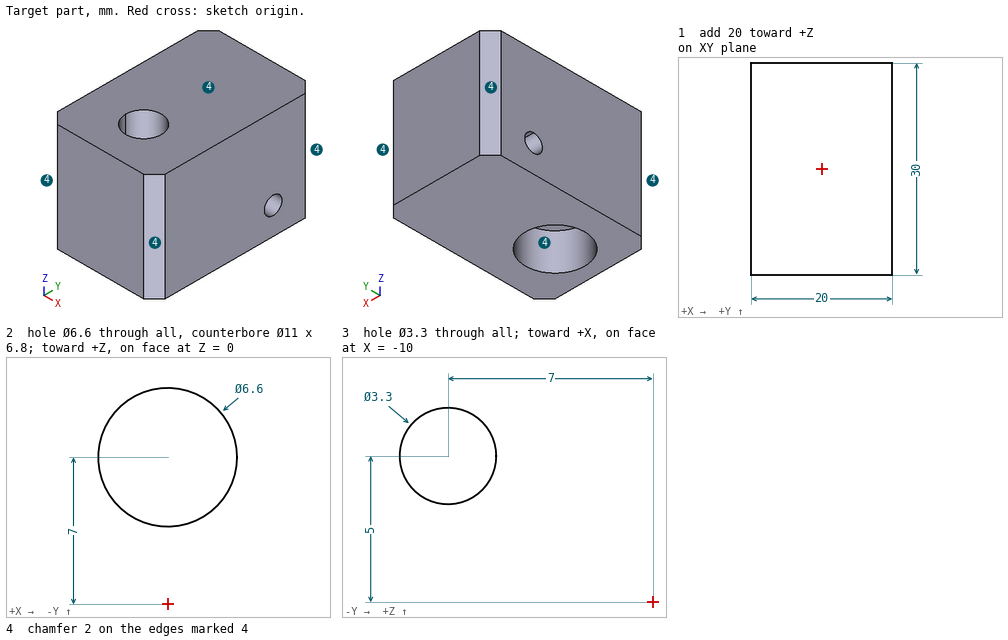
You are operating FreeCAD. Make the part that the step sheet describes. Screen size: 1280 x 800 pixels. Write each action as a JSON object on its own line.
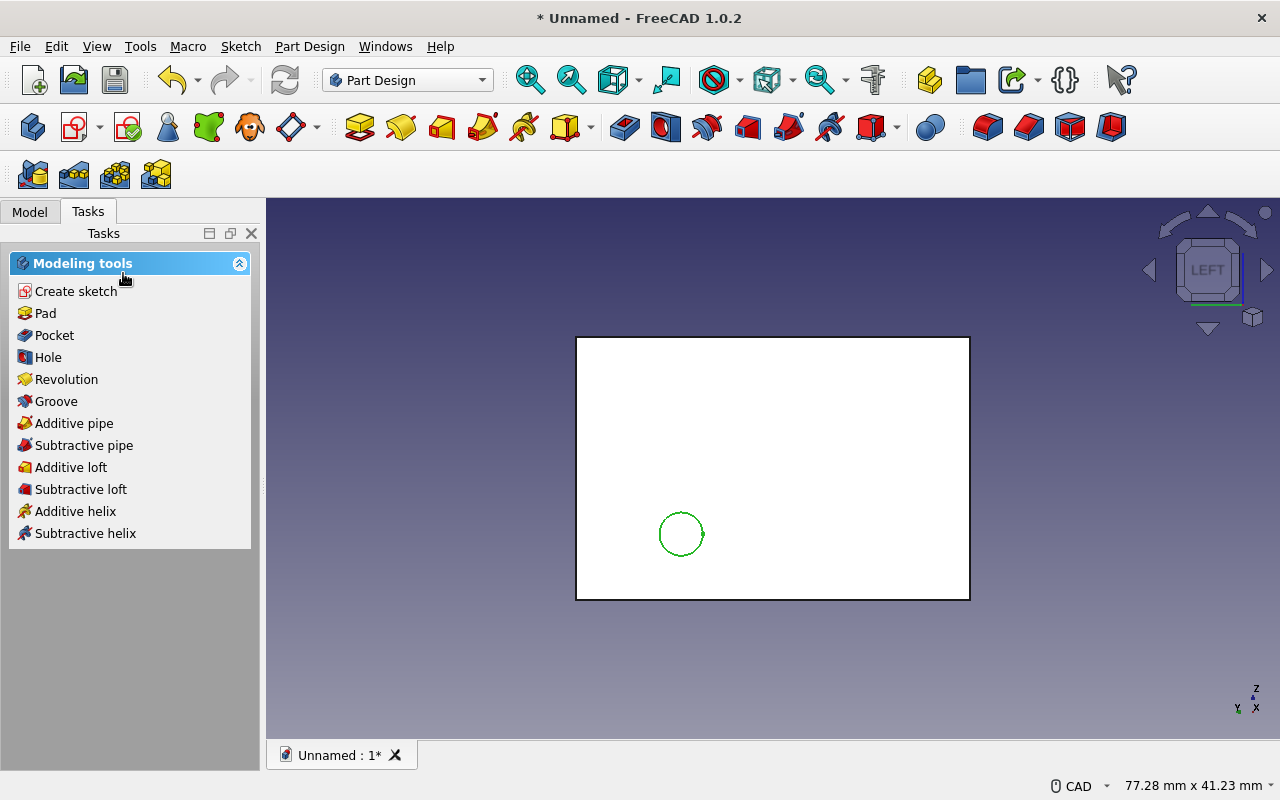
{"action": "left_click", "coordinate": [666, 128]}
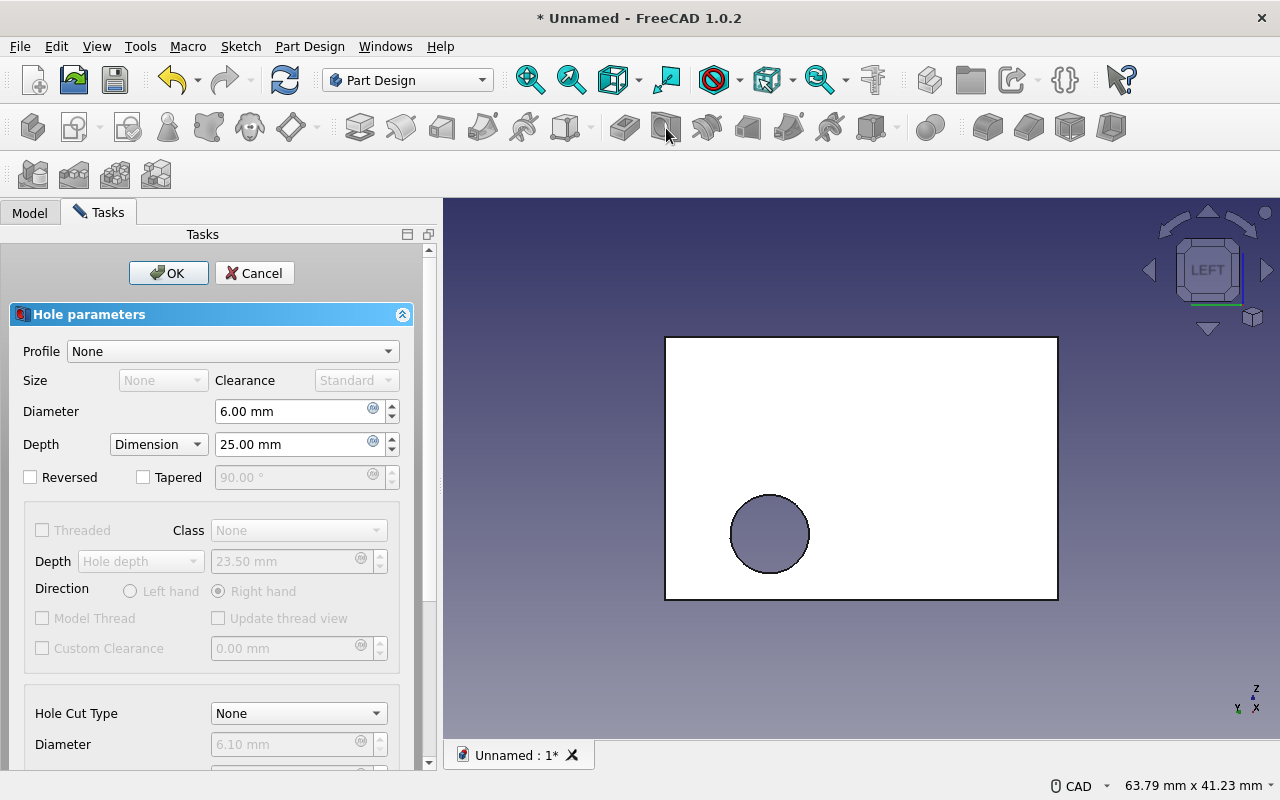
{"action": "triple_click", "coordinate": [300, 412]}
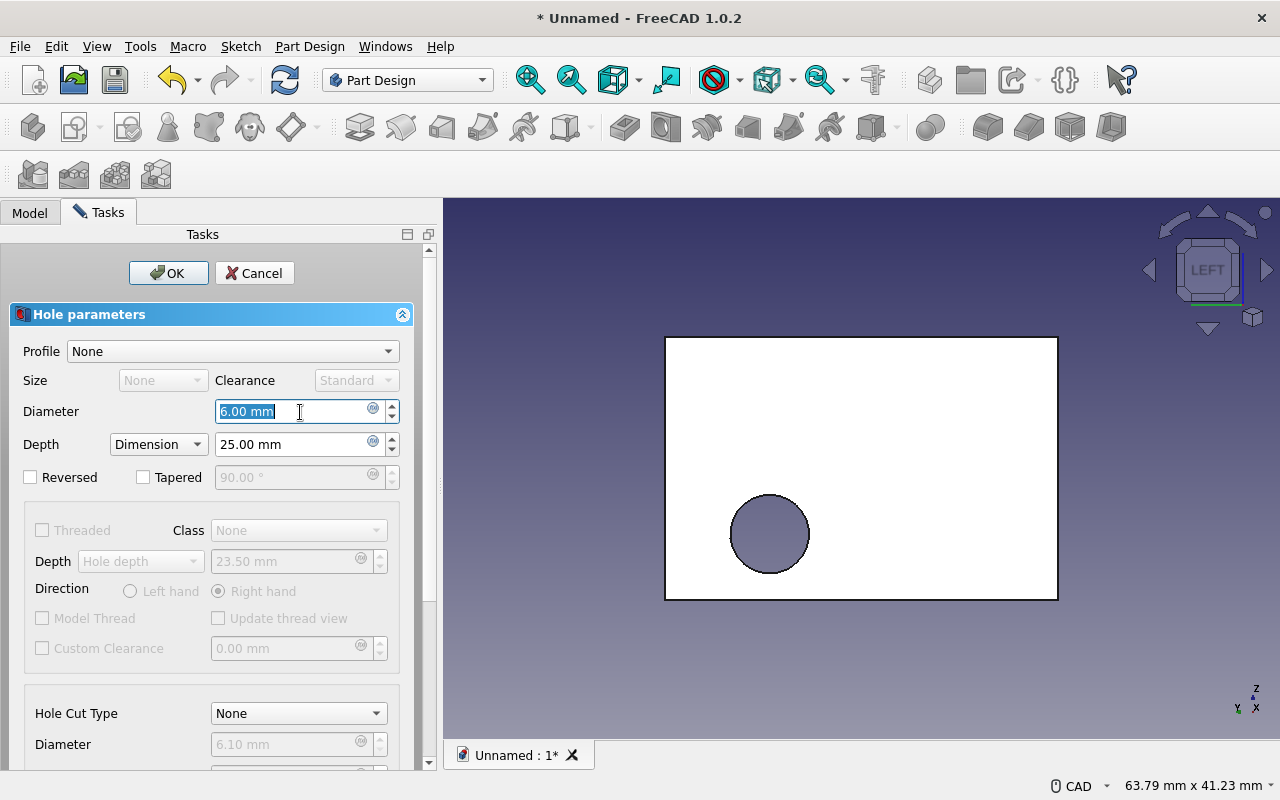
{"action": "type", "text": "3.3"}
{"action": "key", "text": "Tab"}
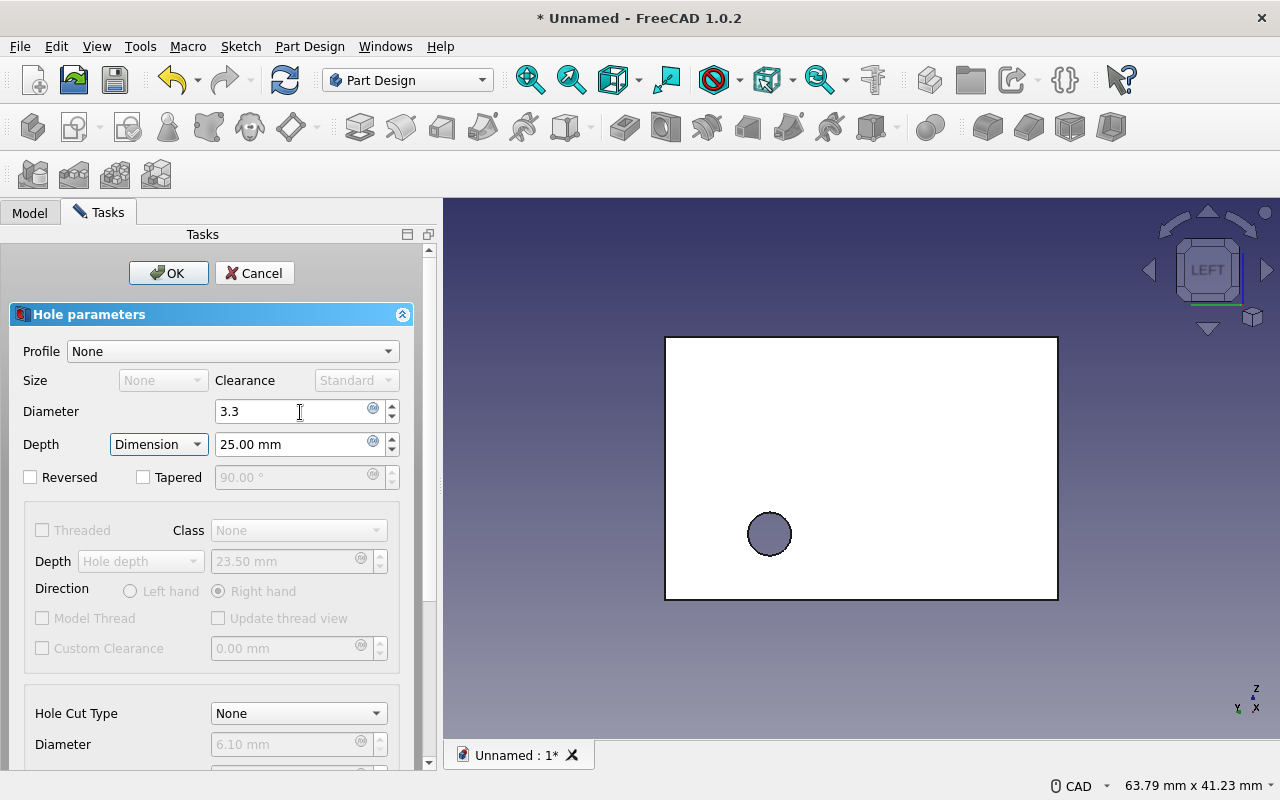
{"action": "left_click", "coordinate": [160, 444]}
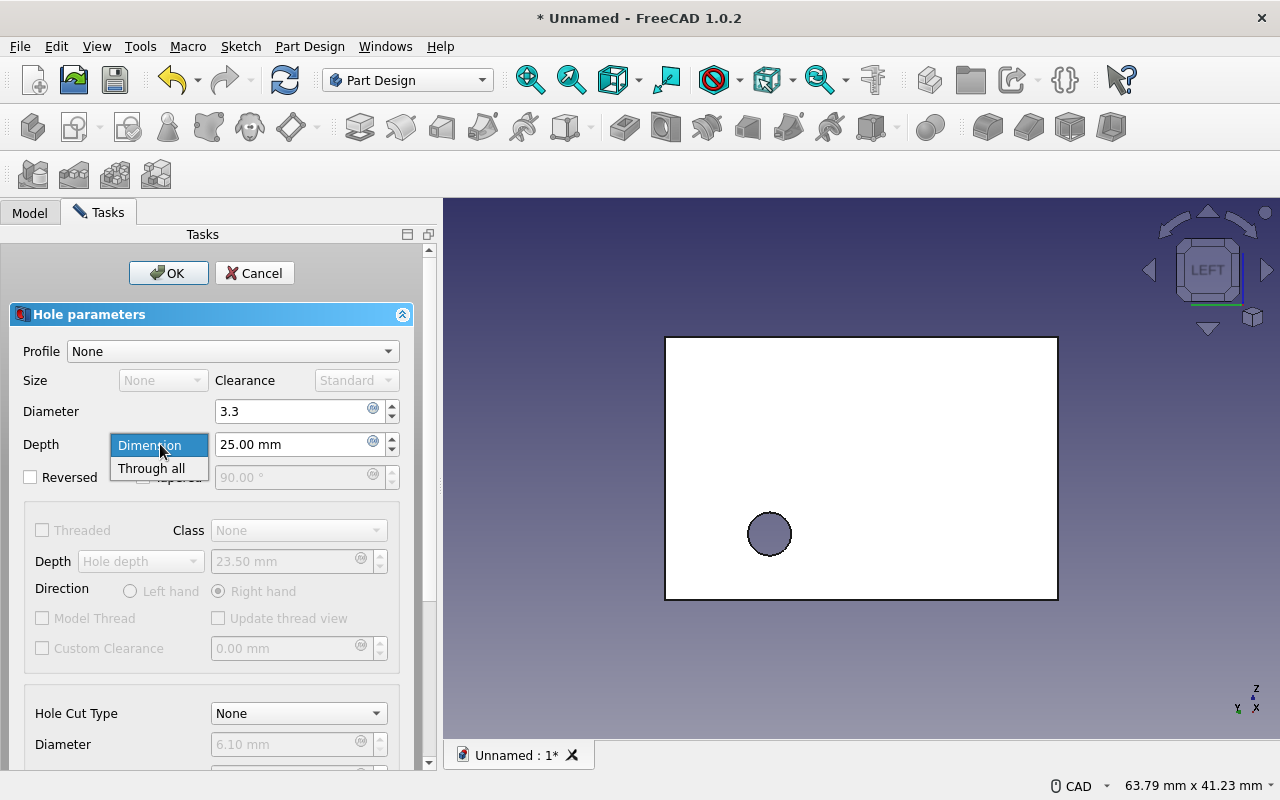
{"action": "left_click", "coordinate": [158, 468]}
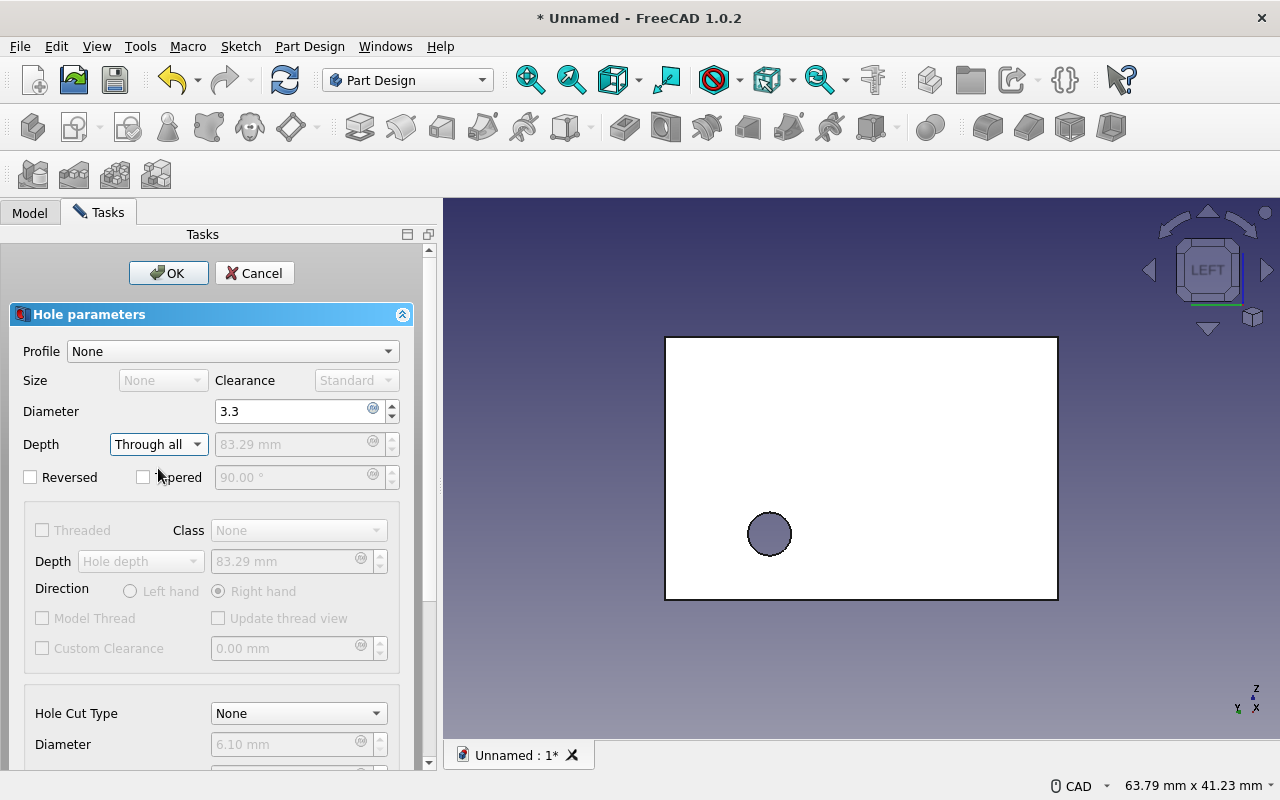
{"action": "left_click", "coordinate": [169, 273]}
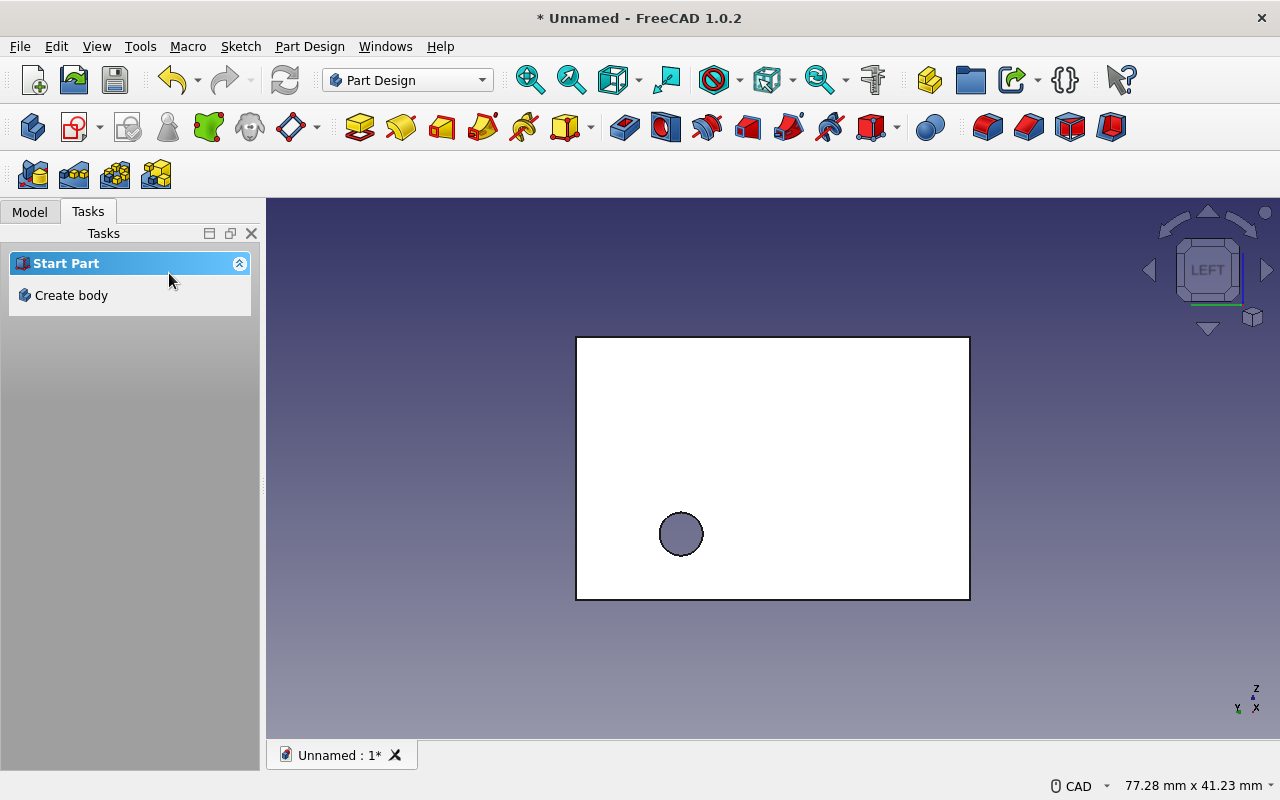
{"action": "left_click", "coordinate": [970, 467]}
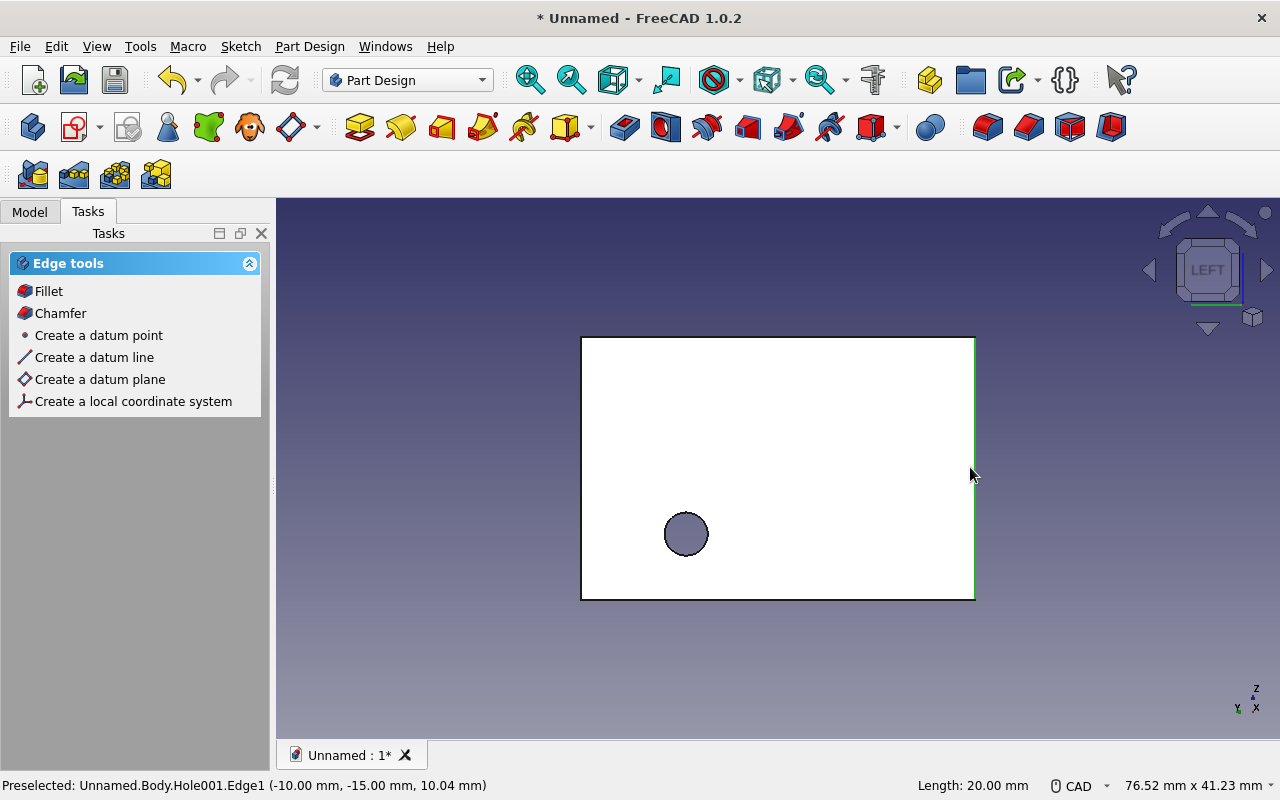
{"action": "left_click", "coordinate": [581, 467], "text": "ctrl"}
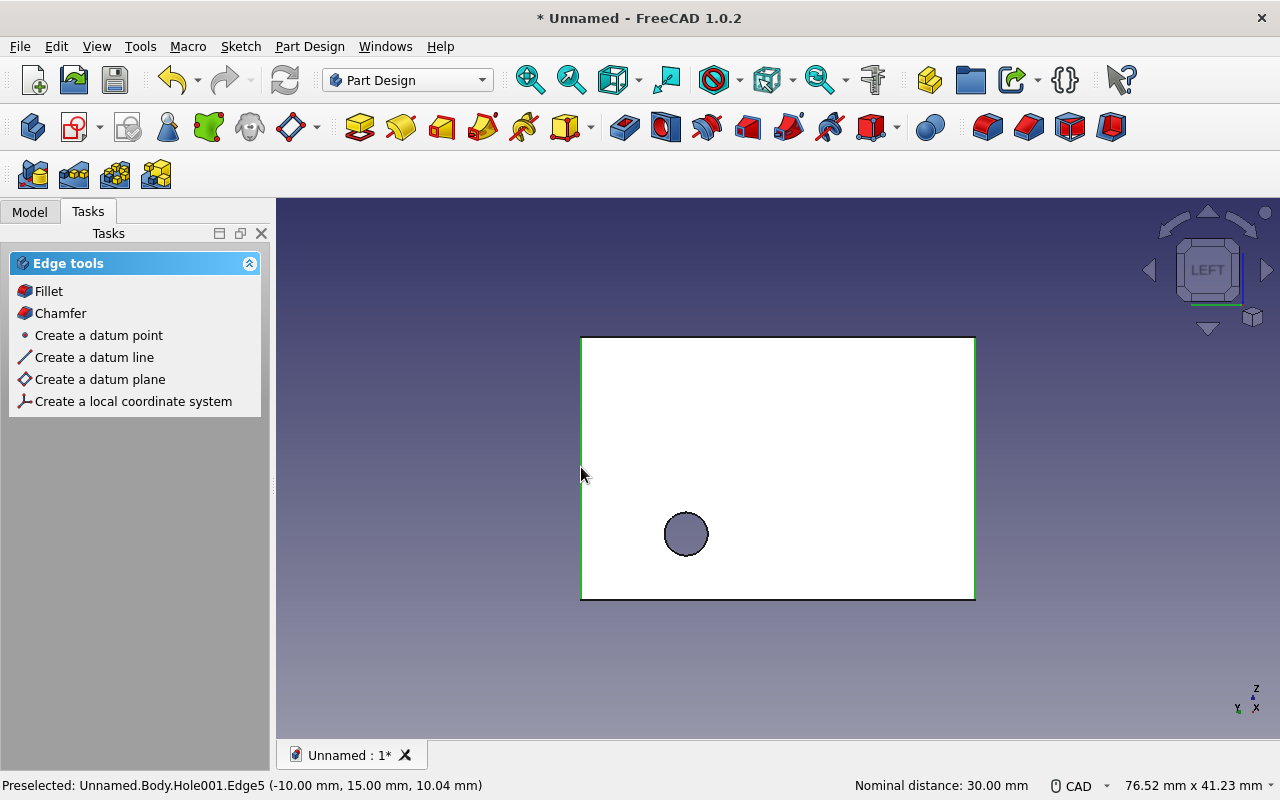
{"action": "key", "text": "0"}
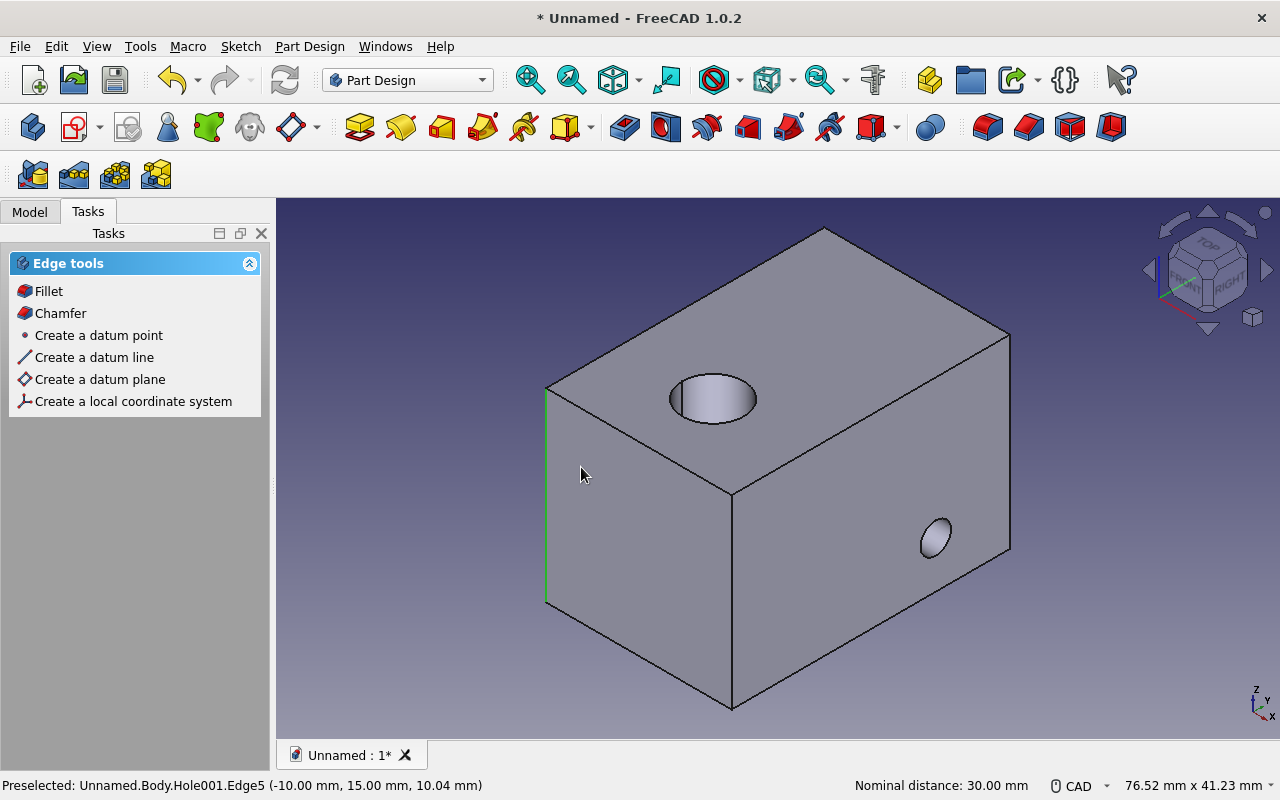
{"action": "left_click", "coordinate": [732, 601], "text": "ctrl"}